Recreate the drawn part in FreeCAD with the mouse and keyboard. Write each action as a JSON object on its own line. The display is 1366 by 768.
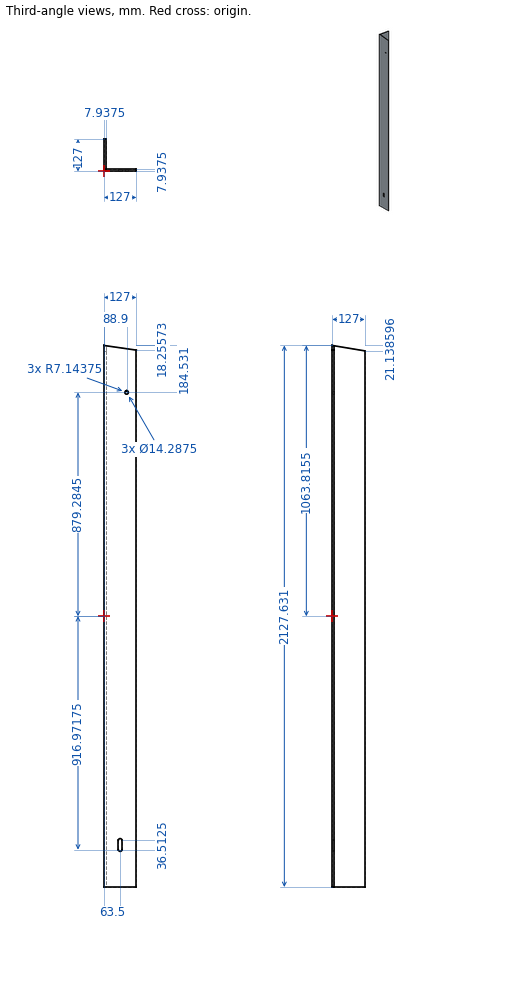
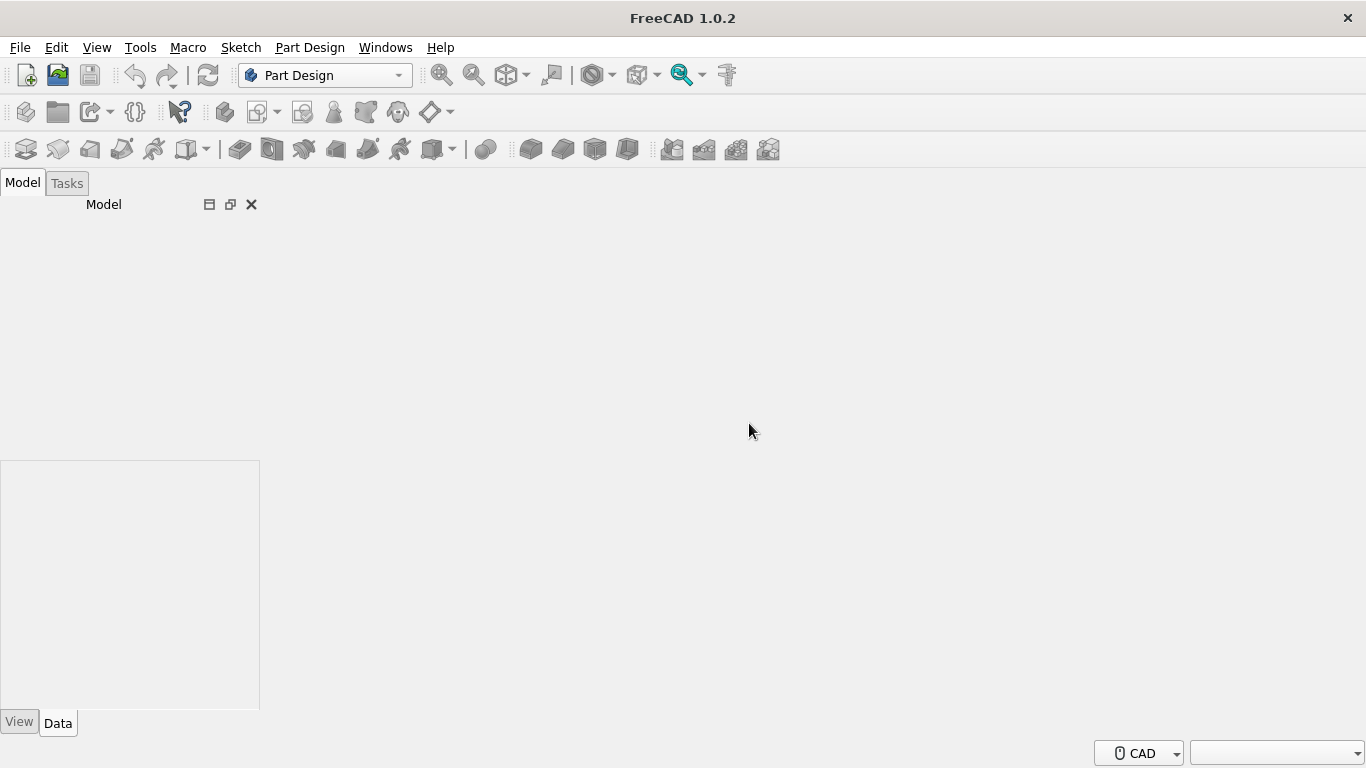
{"action": "key", "text": "ctrl+n"}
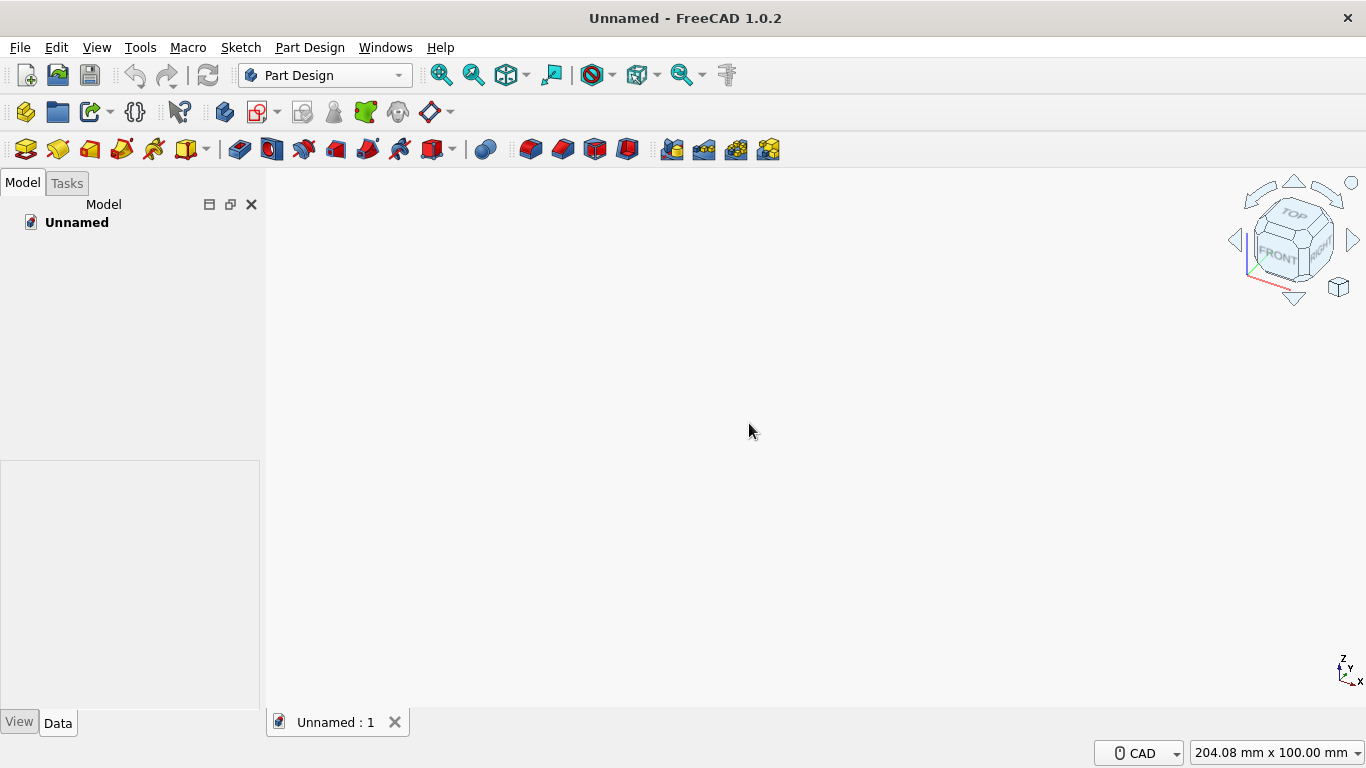
{"action": "left_click", "coordinate": [258, 112]}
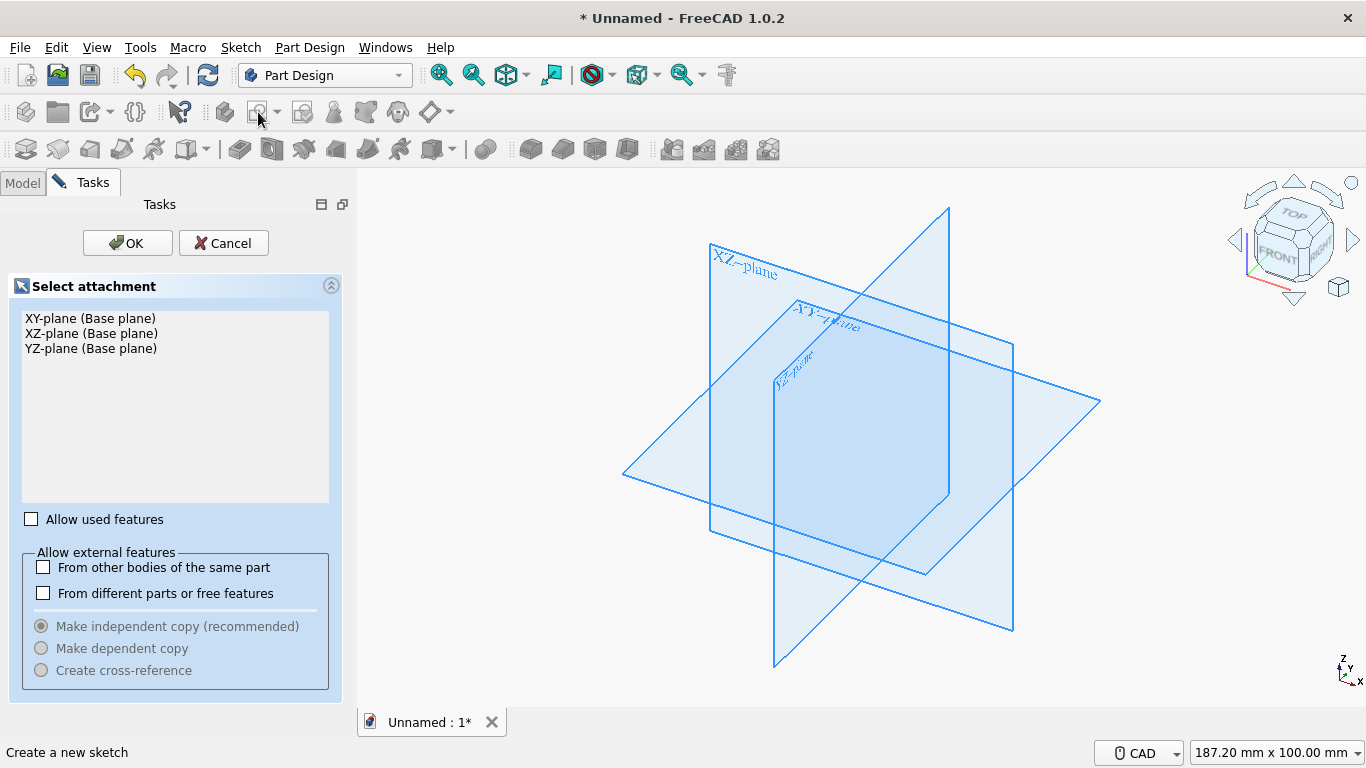
{"action": "left_click", "coordinate": [82, 318]}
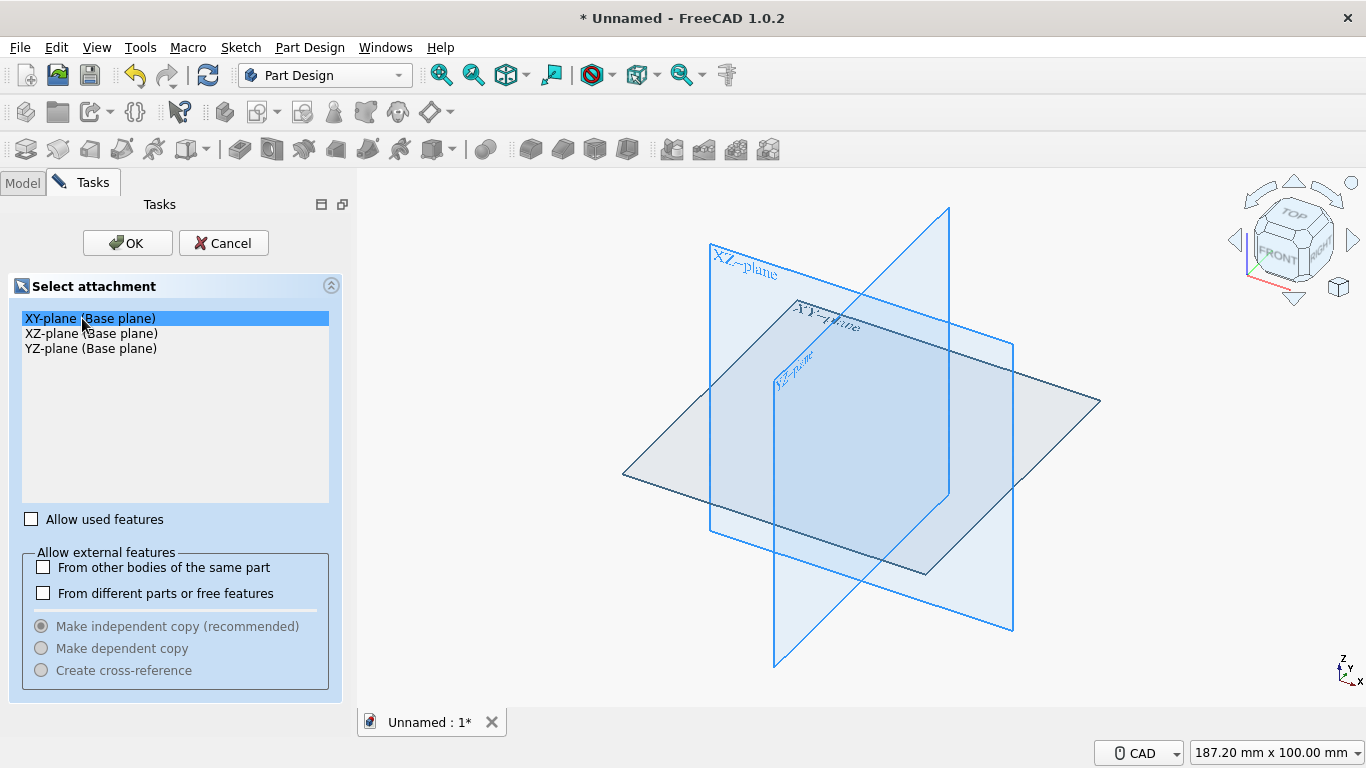
{"action": "left_click", "coordinate": [128, 243]}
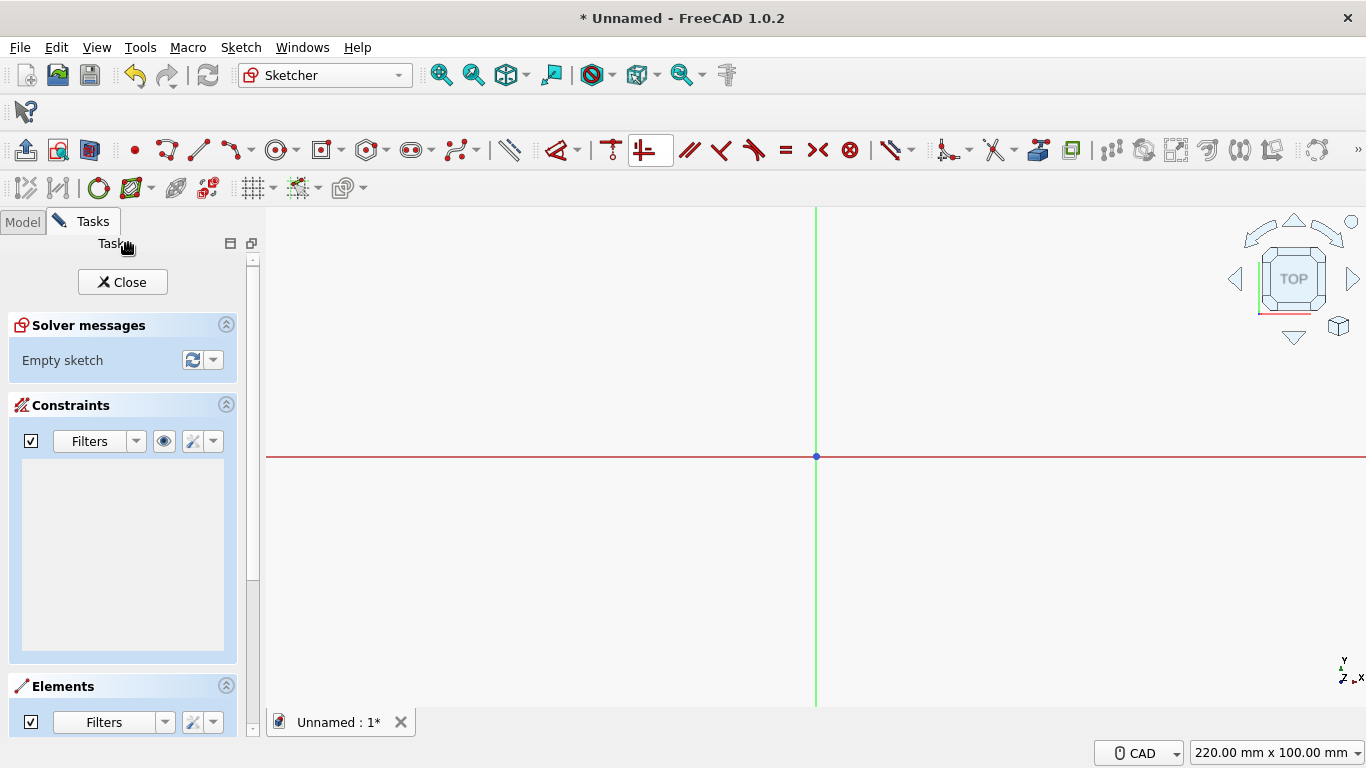
{"action": "scroll", "coordinate": [433, 679], "scroll_direction": "down", "scroll_amount": 4}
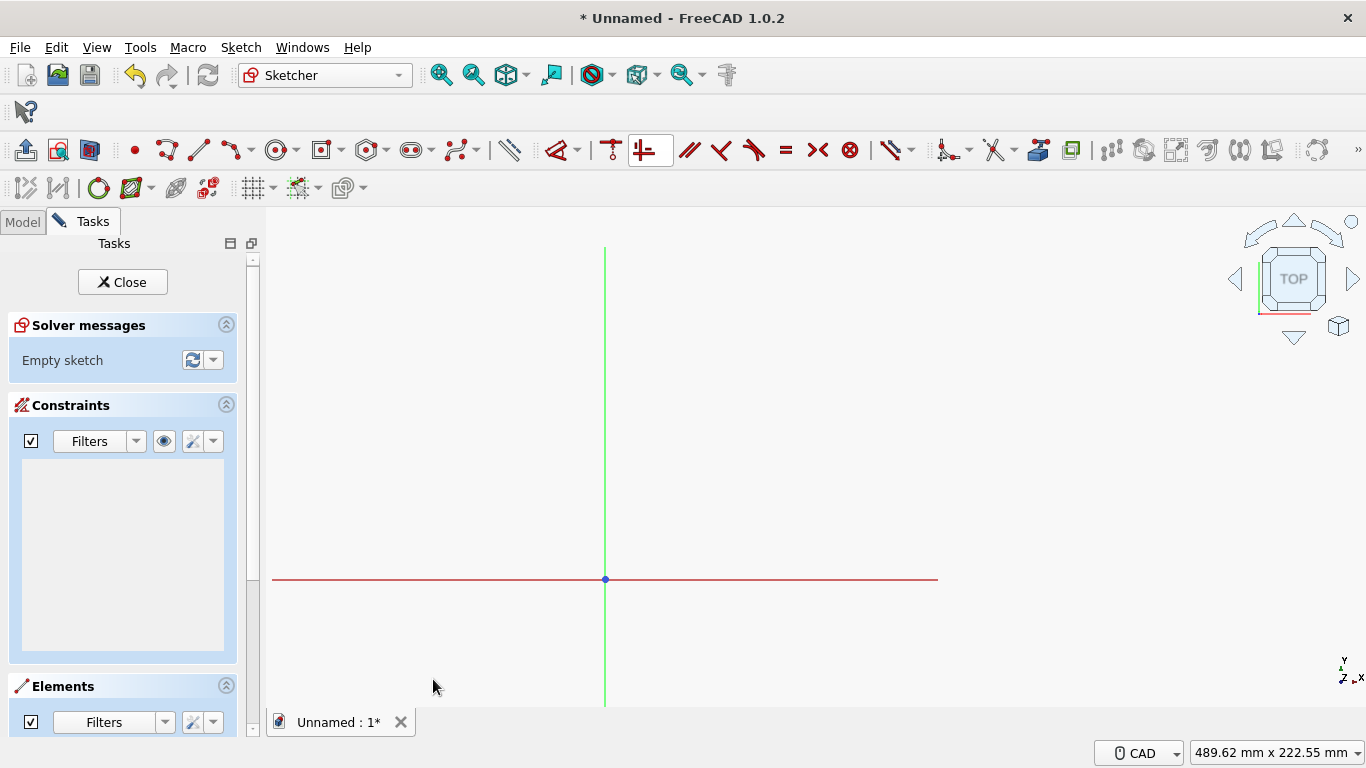
{"action": "key", "text": "g m"}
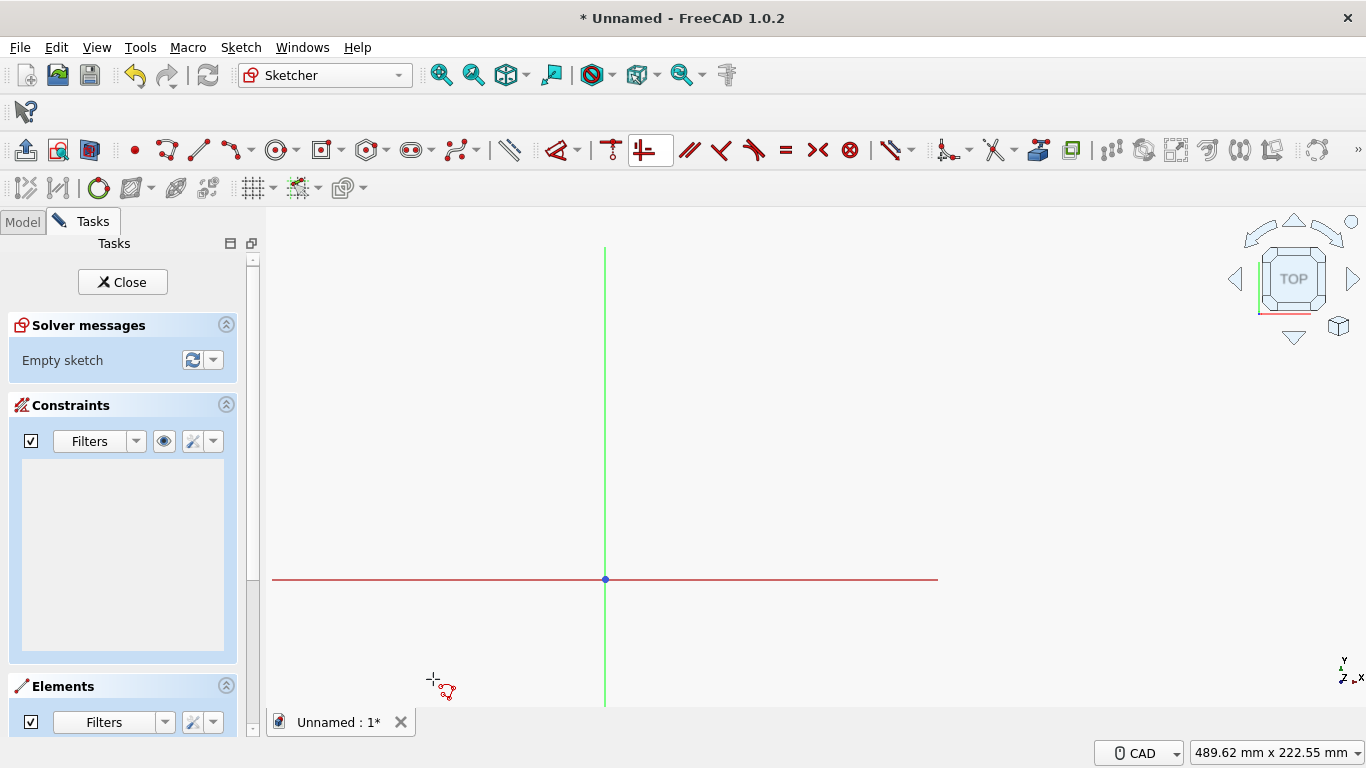
{"action": "left_click", "coordinate": [605, 580]}
{"action": "left_click", "coordinate": [891, 571]}
{"action": "left_click", "coordinate": [891, 562]}
{"action": "left_click", "coordinate": [623, 562]}
{"action": "left_click", "coordinate": [623, 294]}
{"action": "left_click", "coordinate": [614, 294]}
{"action": "left_click", "coordinate": [605, 580]}
{"action": "key", "text": "Escape"}
{"action": "key", "text": "Escape"}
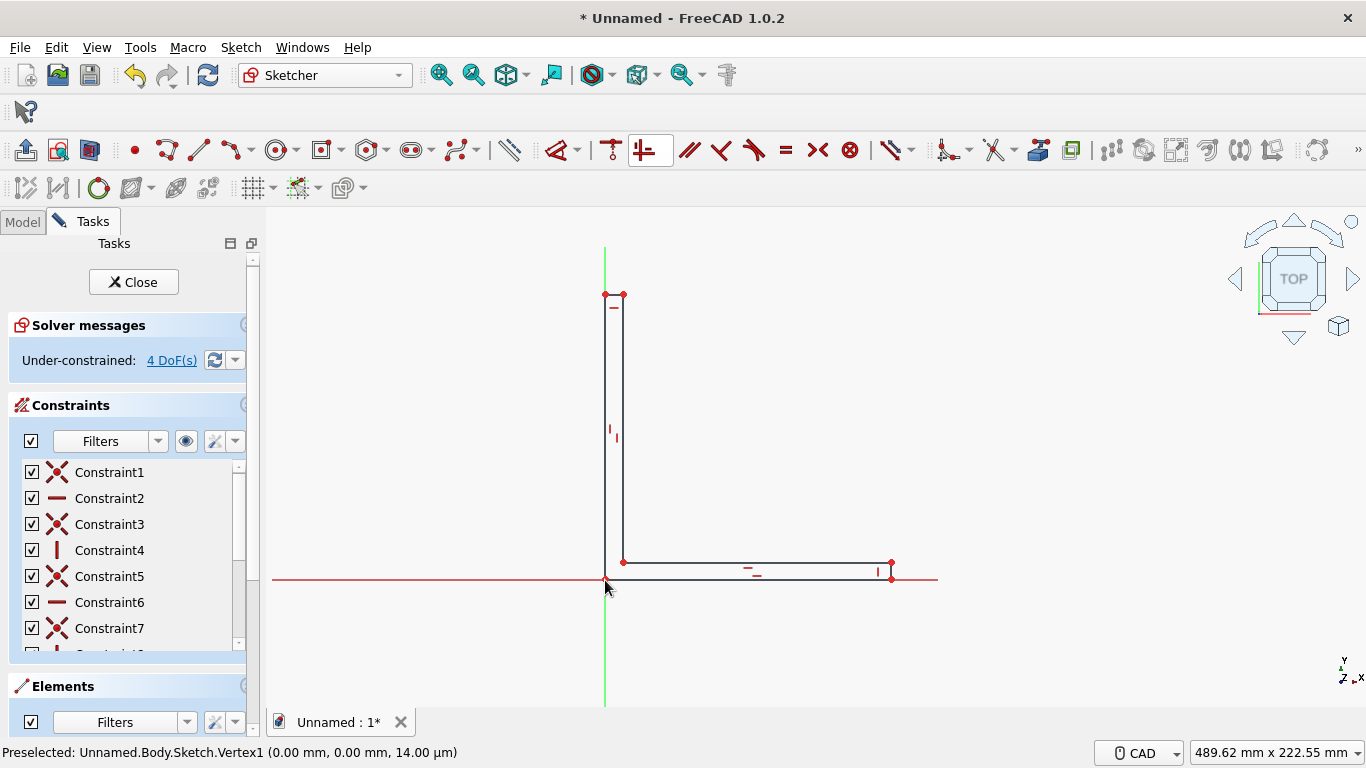
{"action": "key", "text": "d"}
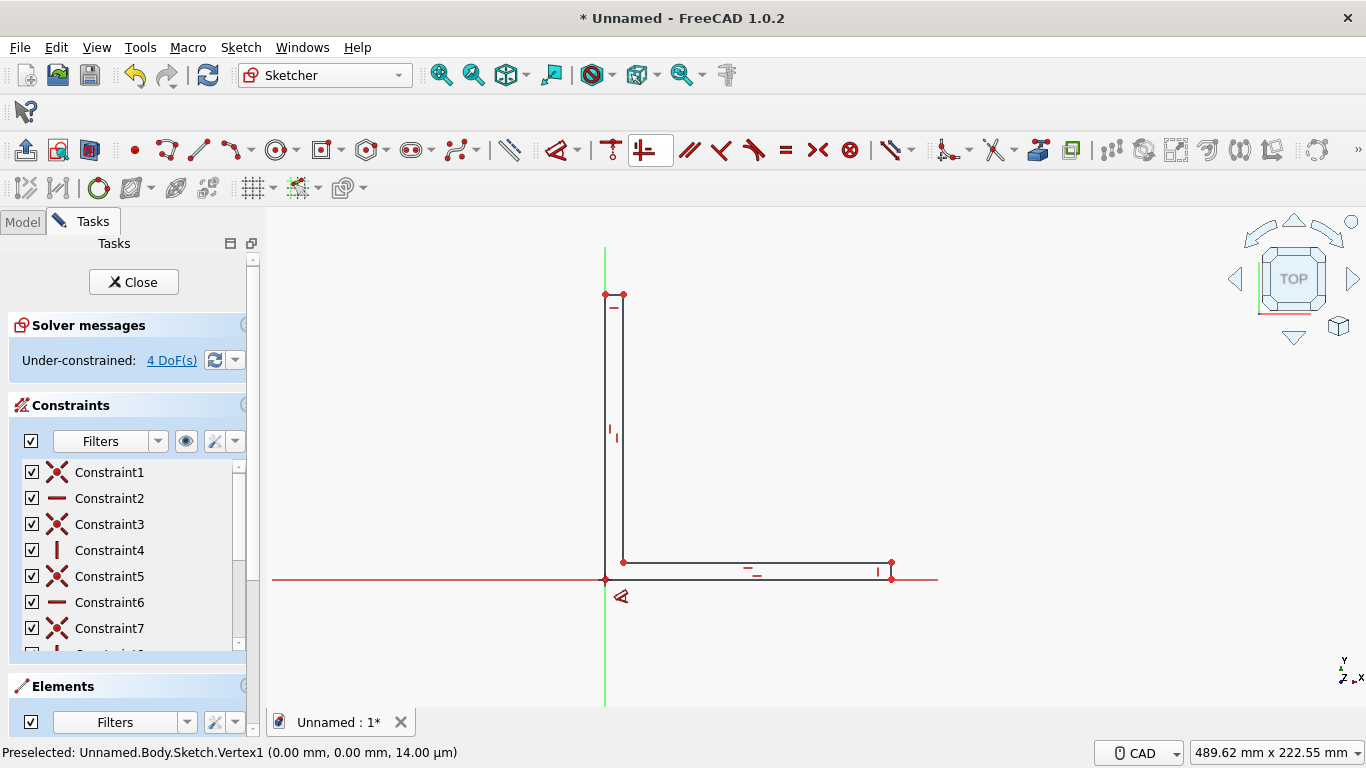
{"action": "left_click", "coordinate": [691, 580]}
{"action": "left_click", "coordinate": [748, 614]}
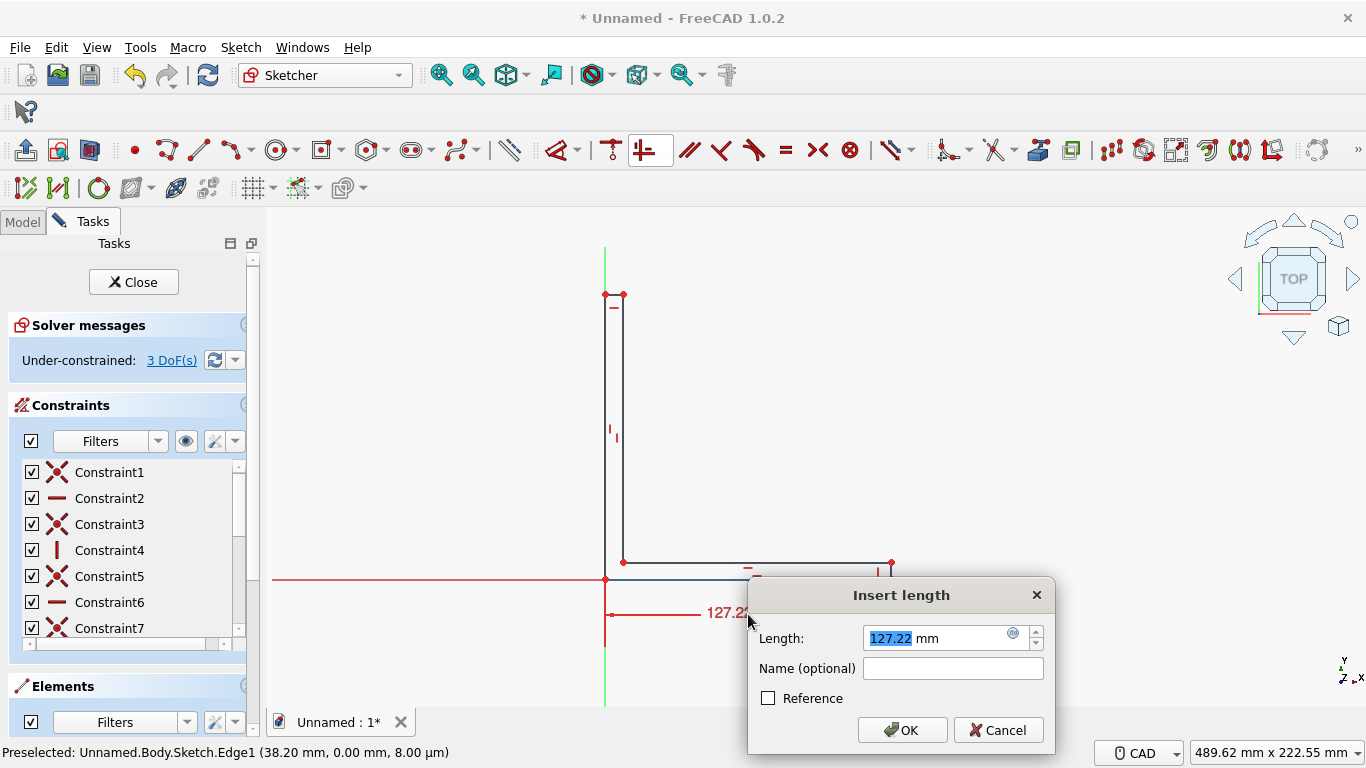
{"action": "type", "text": "127"}
{"action": "key", "text": "Return"}